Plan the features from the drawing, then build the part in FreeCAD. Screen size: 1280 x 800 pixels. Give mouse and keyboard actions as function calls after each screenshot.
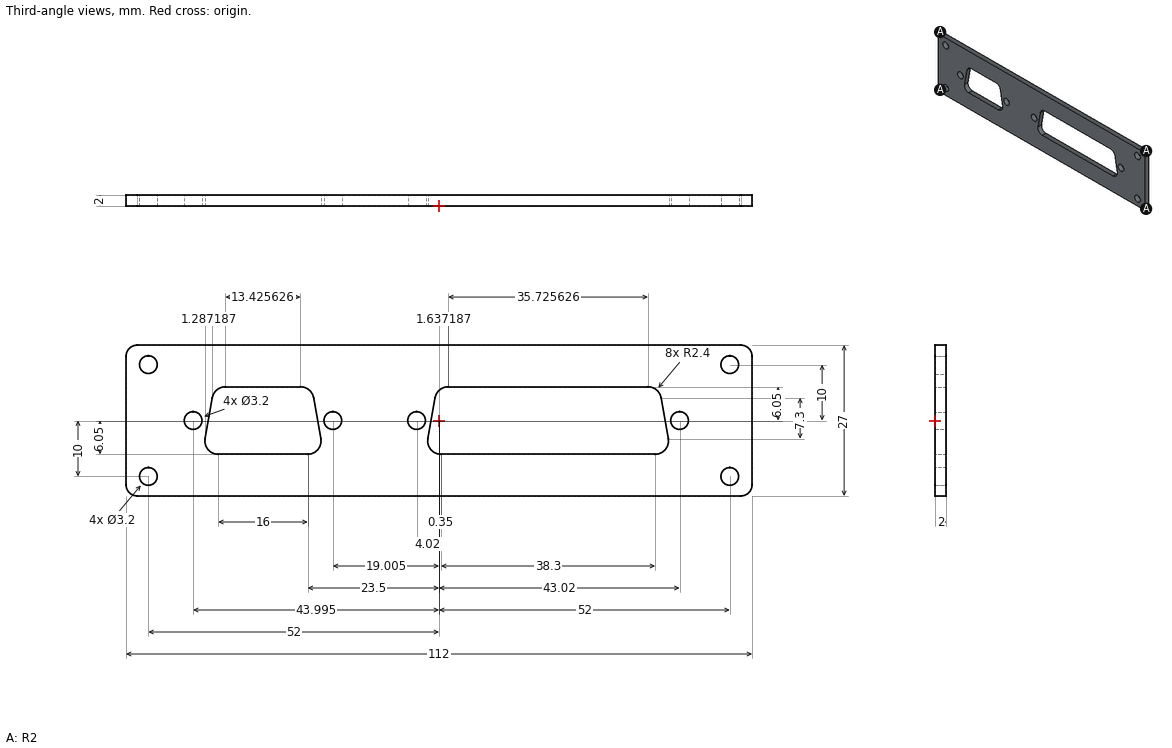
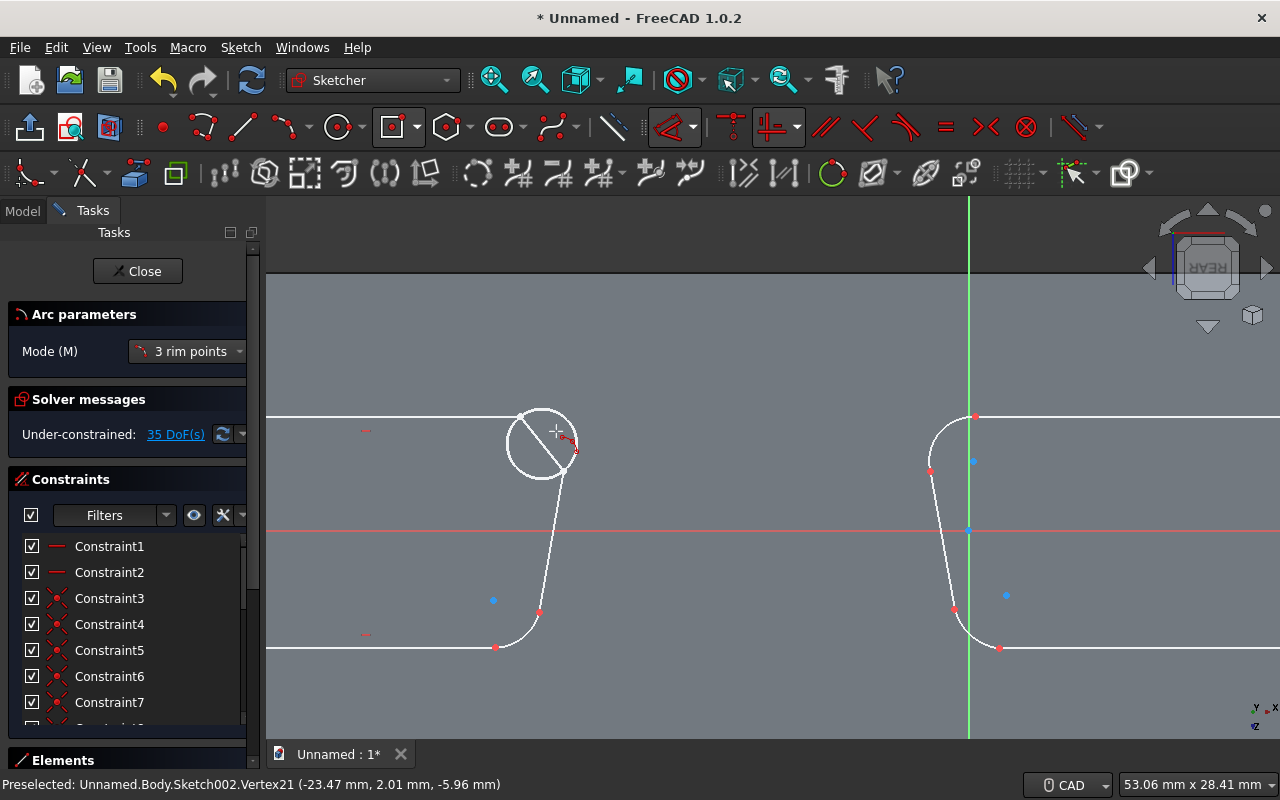
click(555, 431)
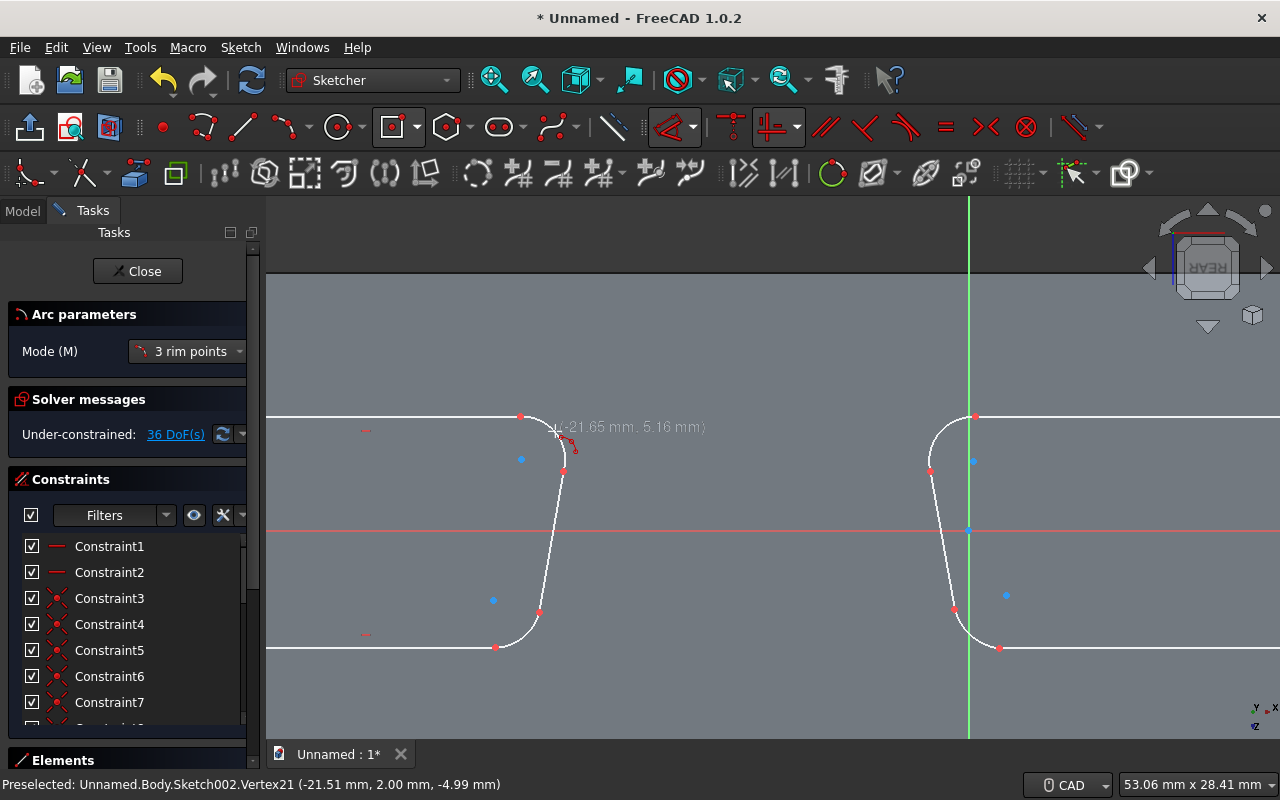
click(338, 128)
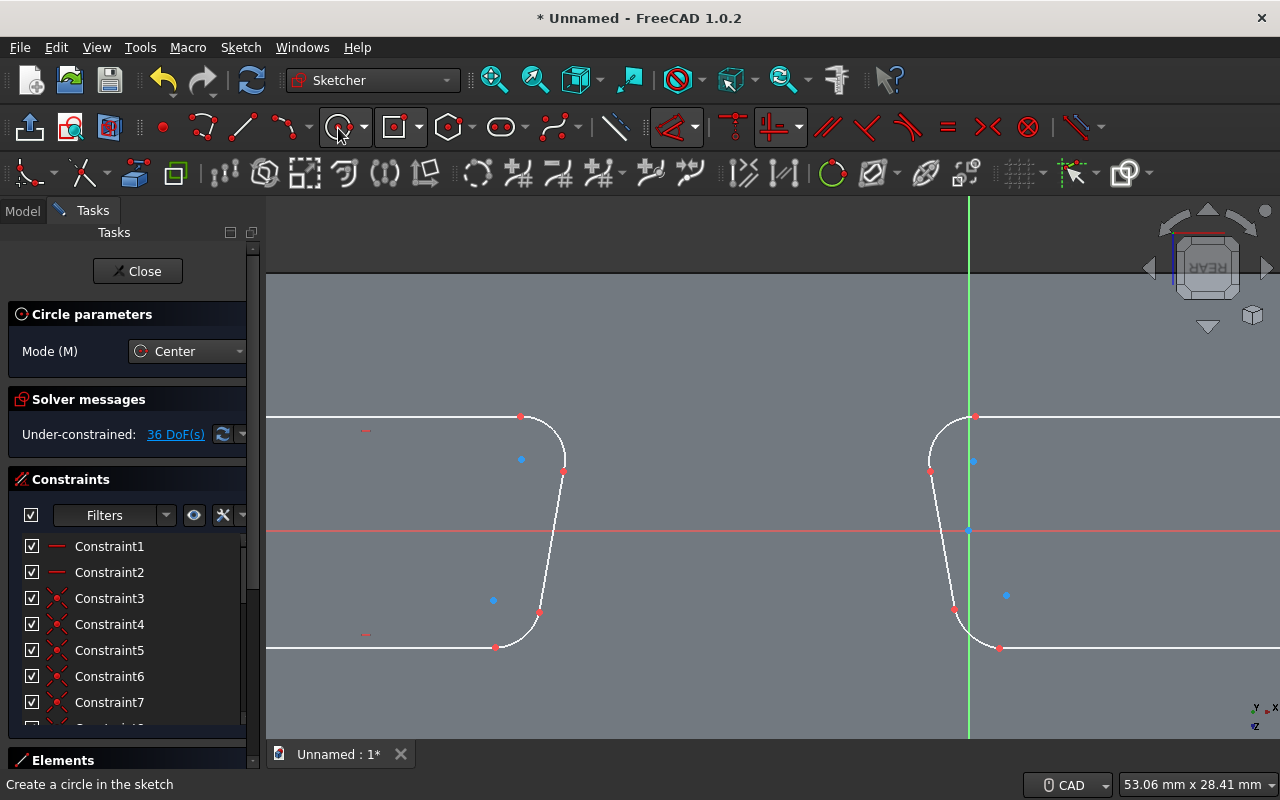
scroll(556, 431, down, 5)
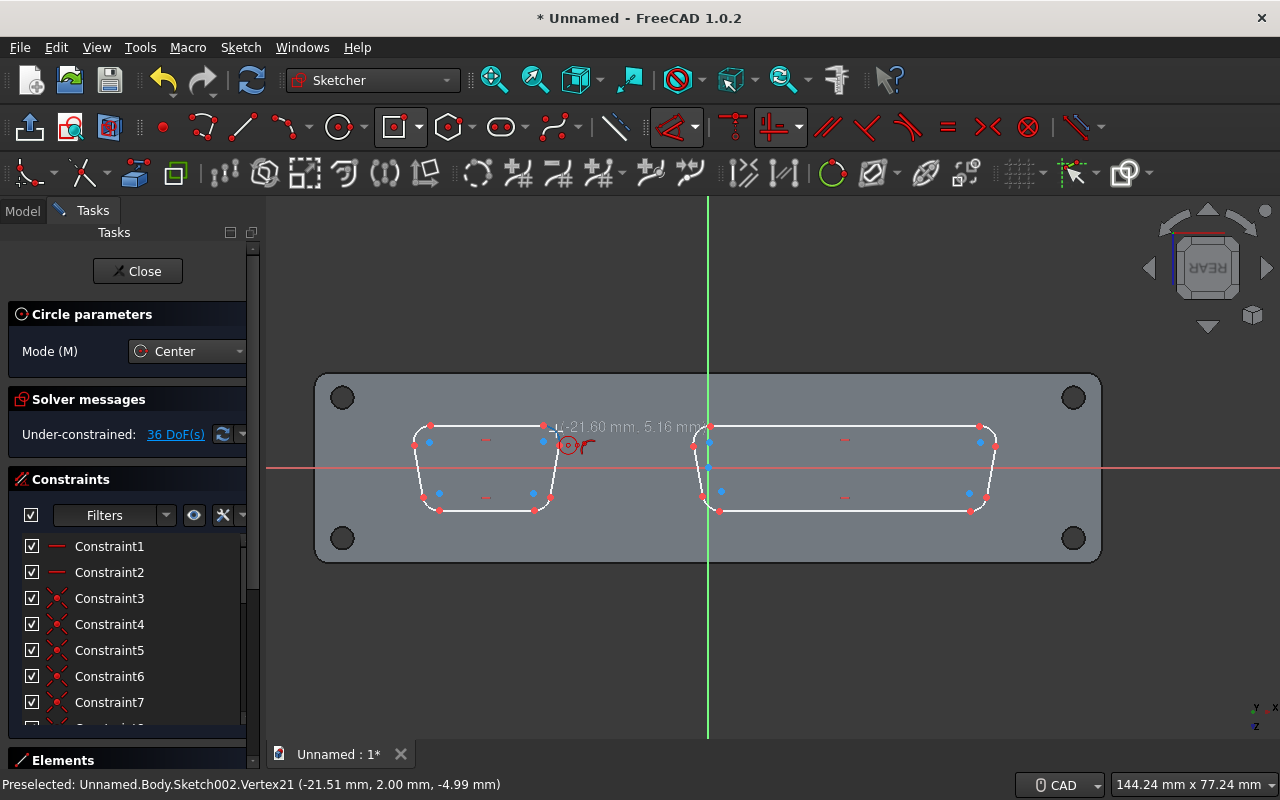
scroll(399, 468, up, 4)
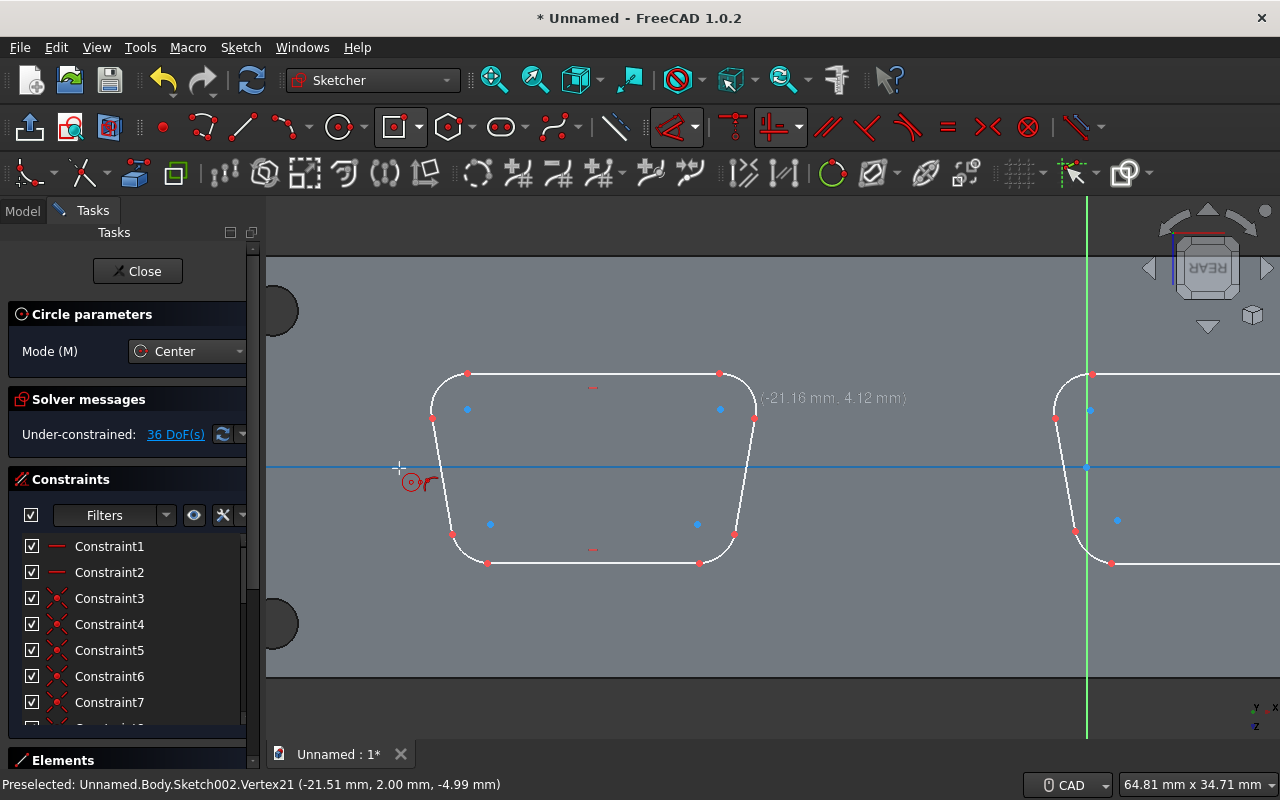
click(398, 467)
click(416, 450)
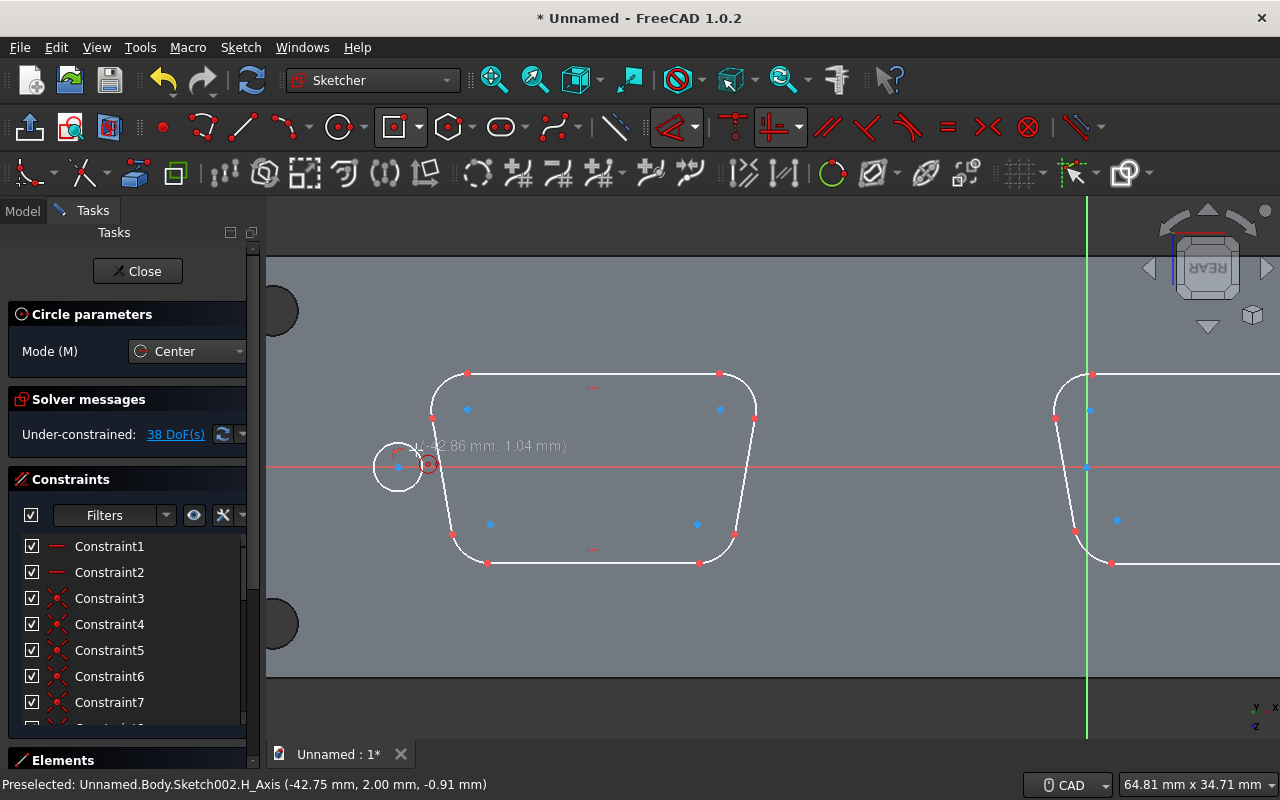
click(789, 467)
click(807, 450)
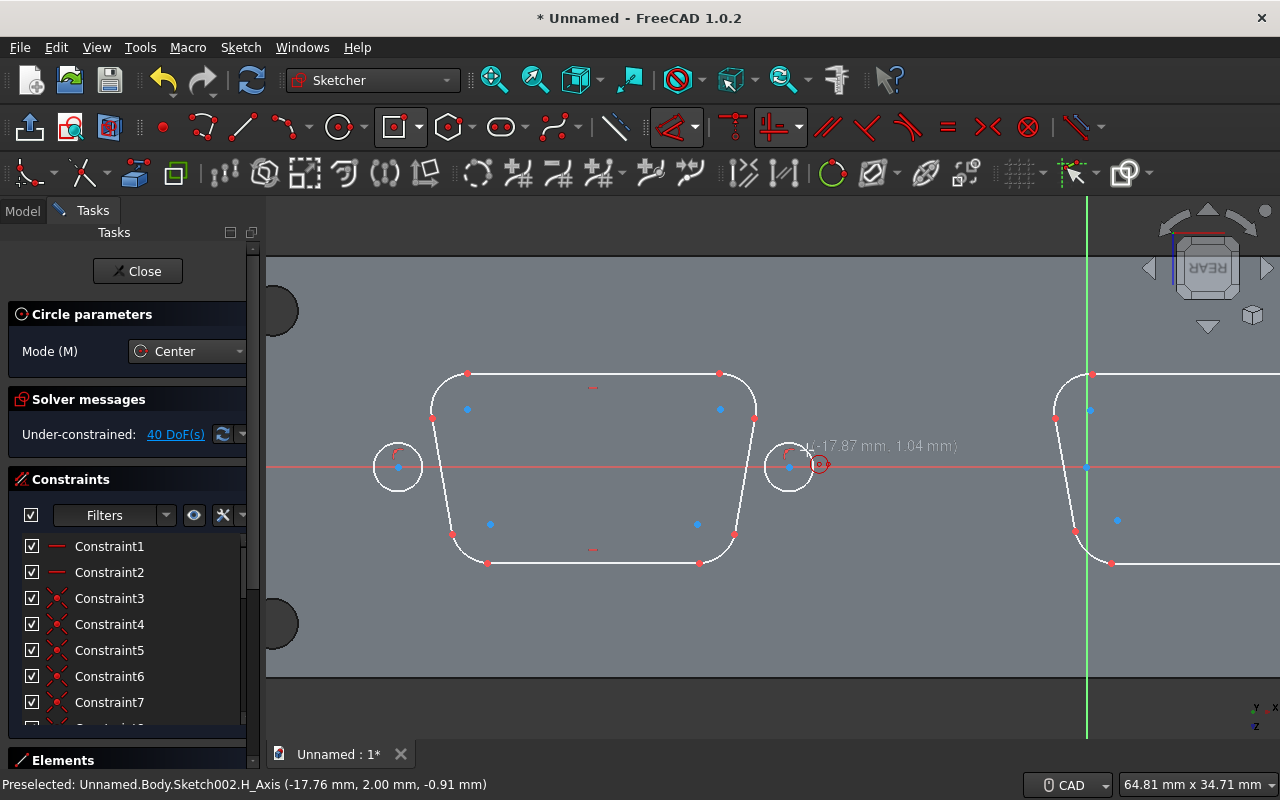
click(1024, 467)
click(1041, 450)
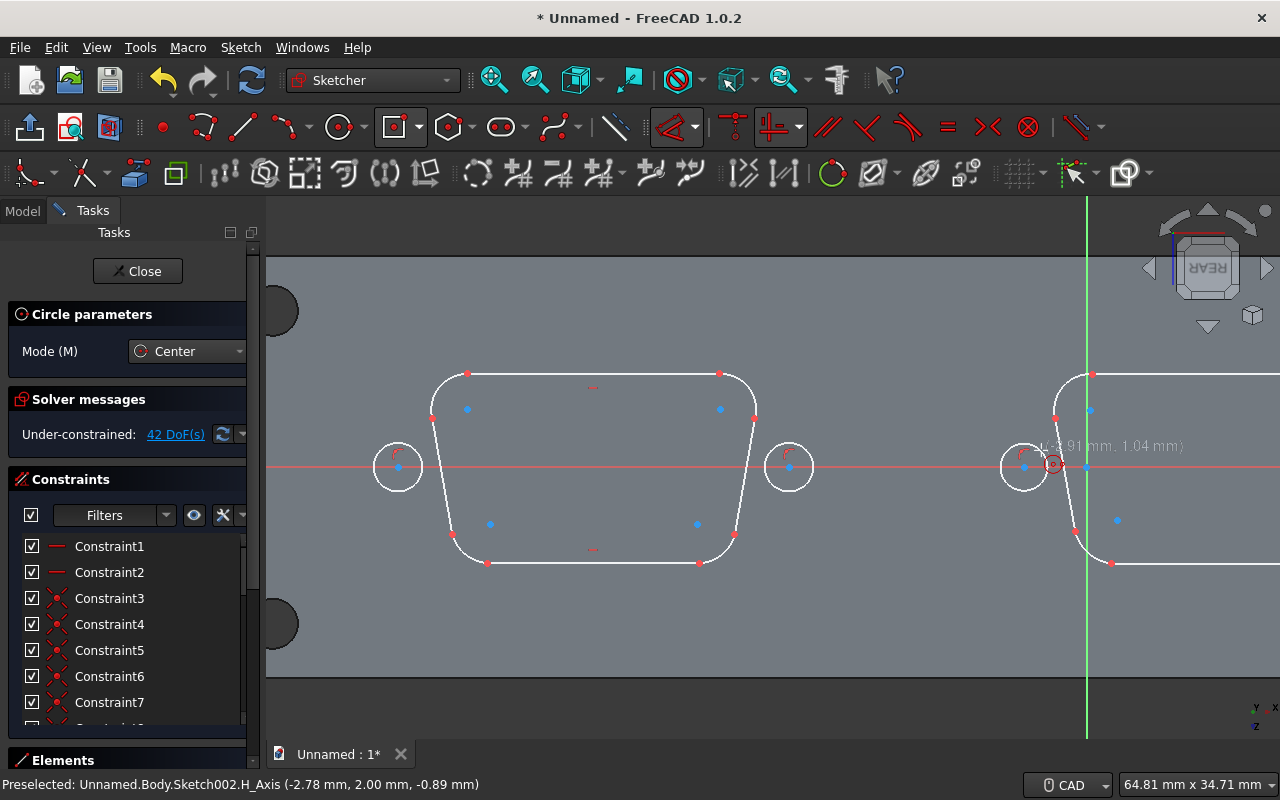
scroll(399, 468, down, 4)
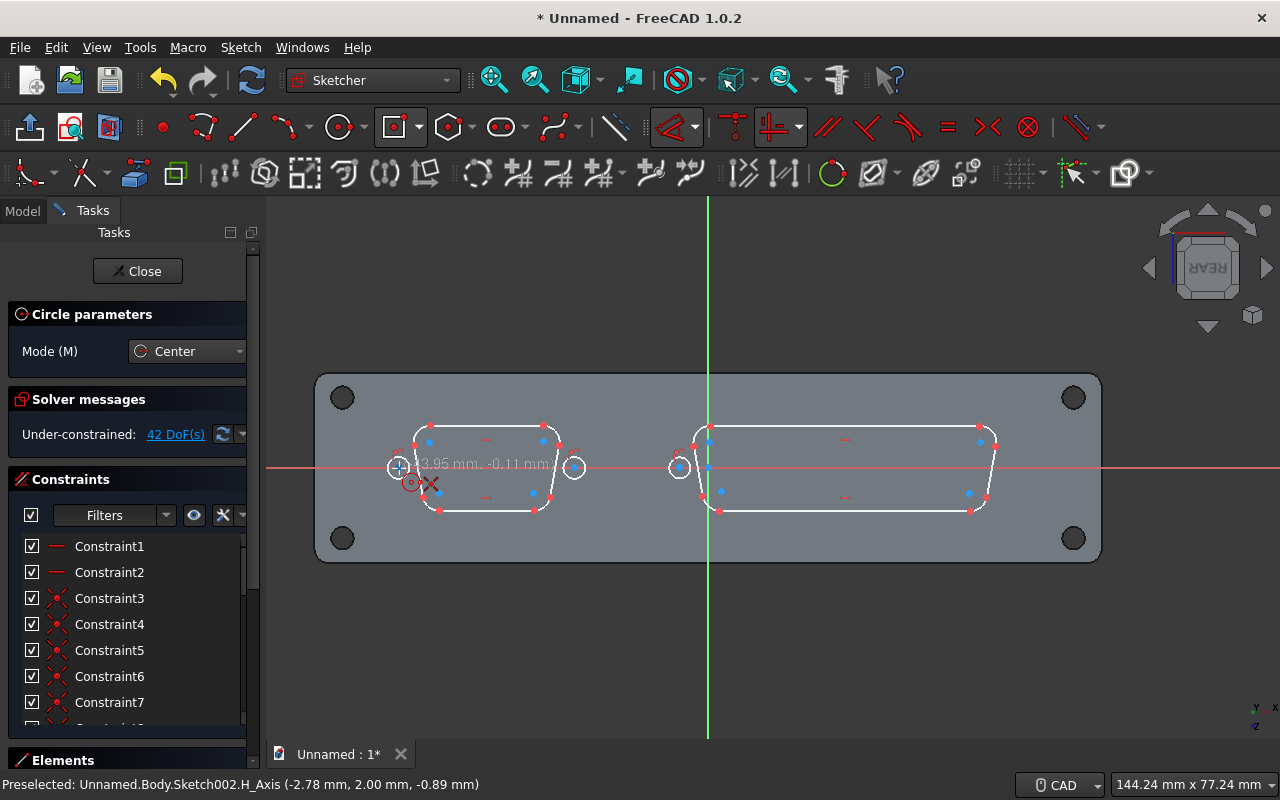
scroll(1010, 468, up, 4)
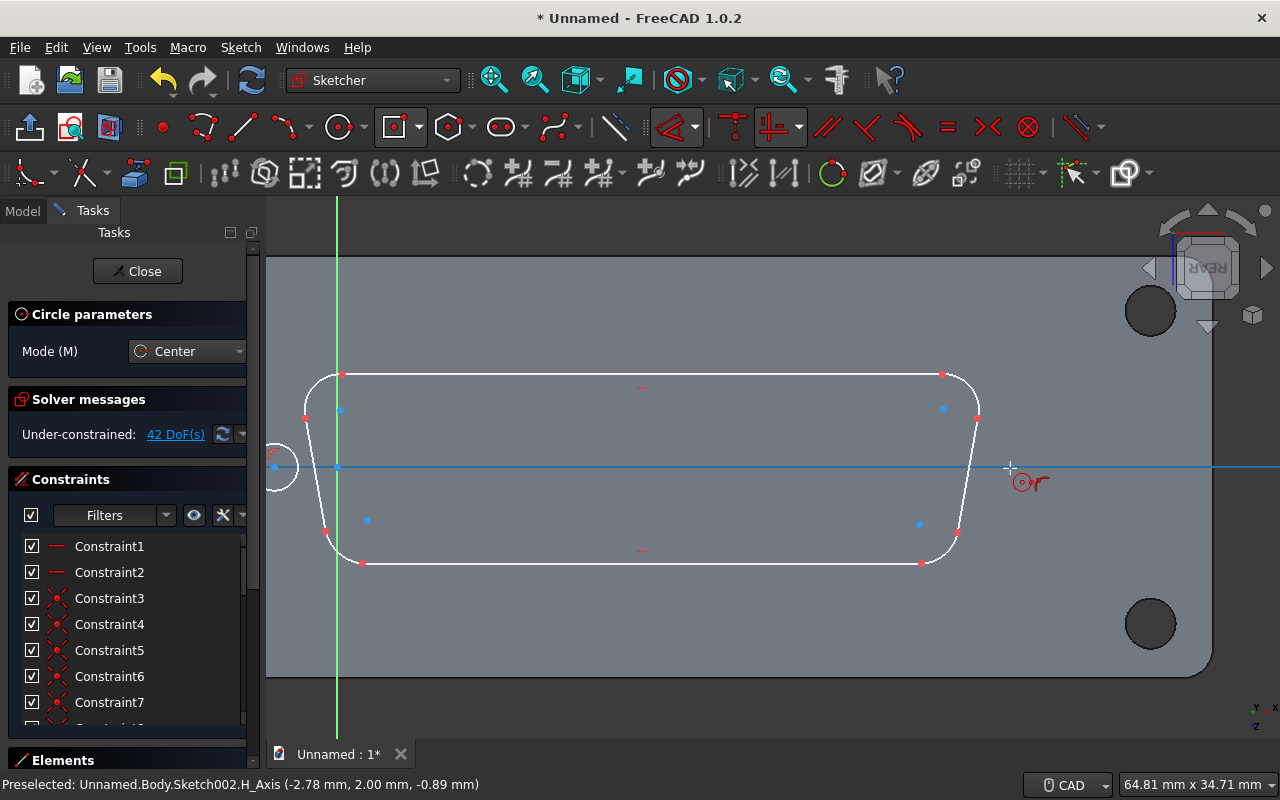
click(1010, 467)
click(1028, 450)
key(Escape)